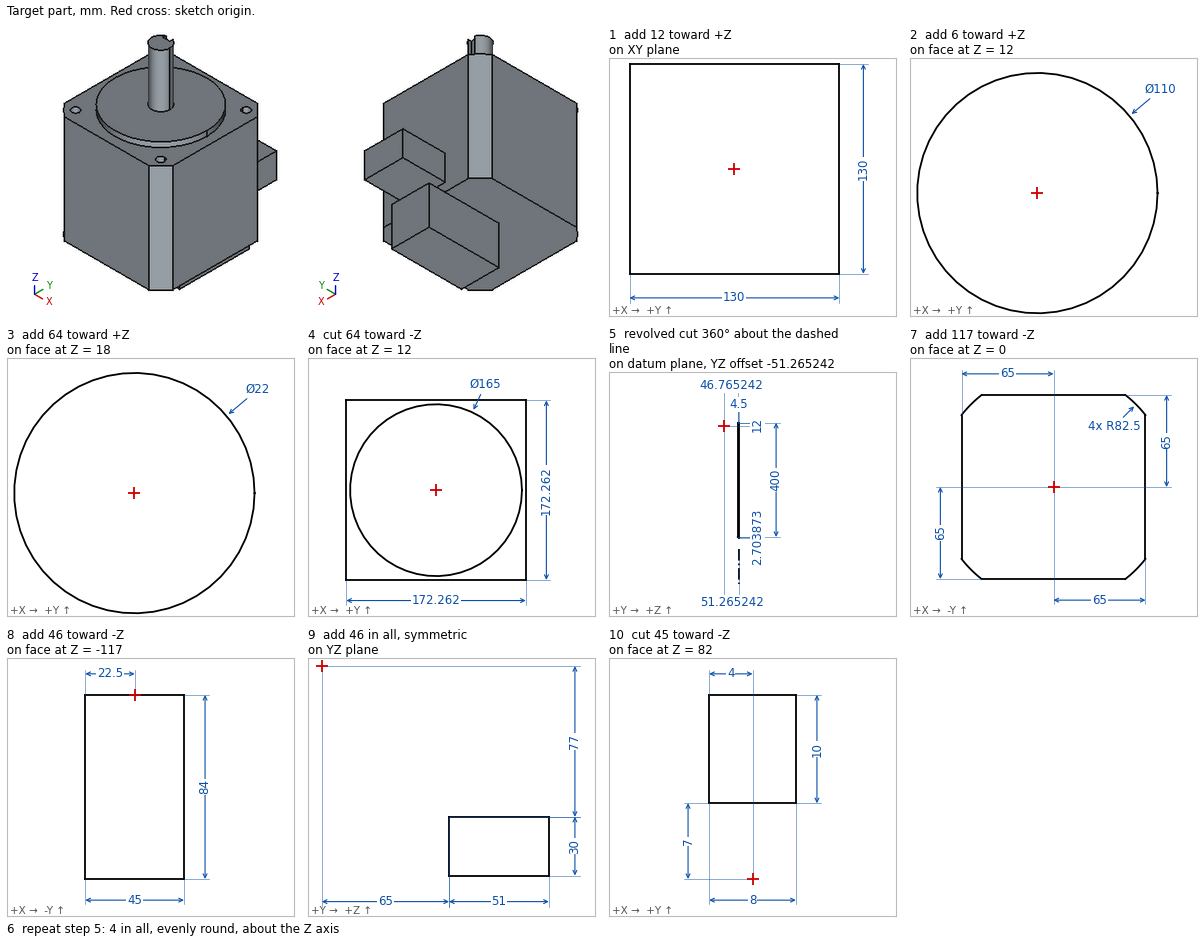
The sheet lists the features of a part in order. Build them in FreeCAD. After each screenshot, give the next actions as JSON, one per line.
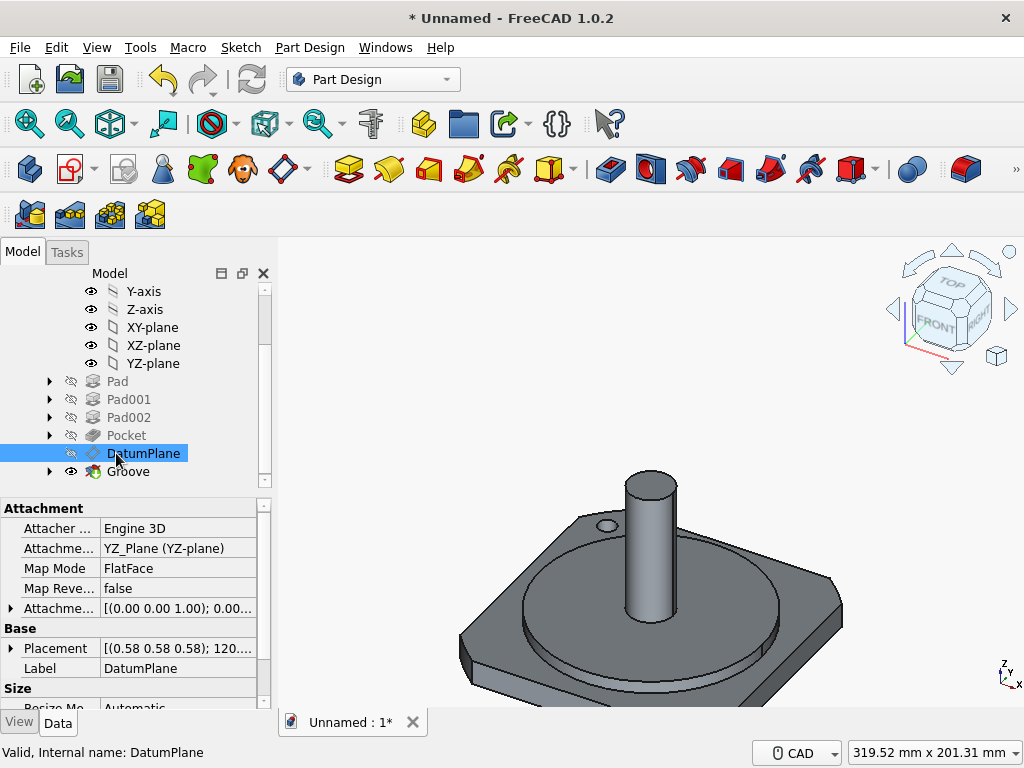
{"action": "left_click", "coordinate": [30, 124]}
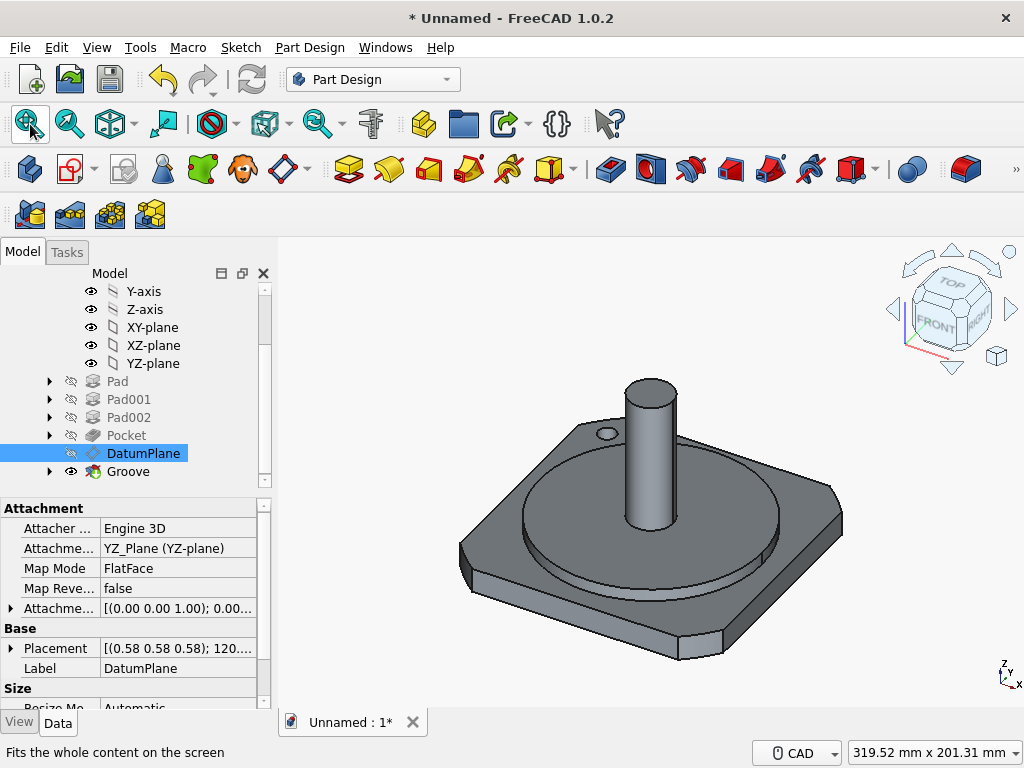
{"action": "left_click", "coordinate": [116, 471]}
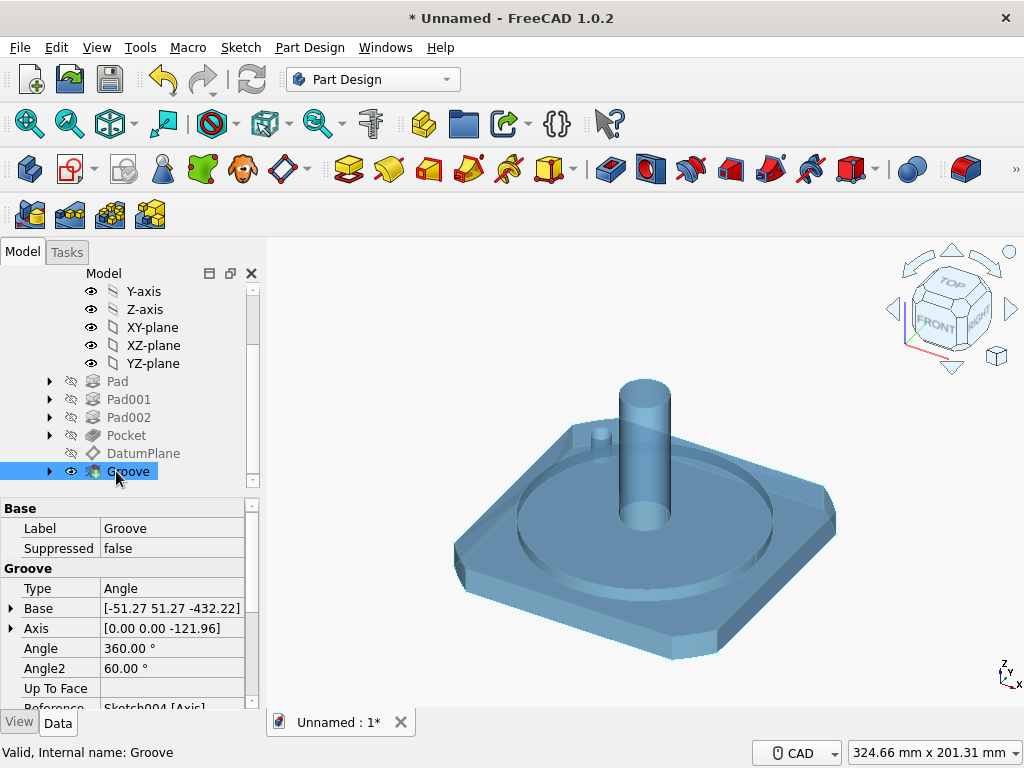
{"action": "left_click", "coordinate": [110, 214]}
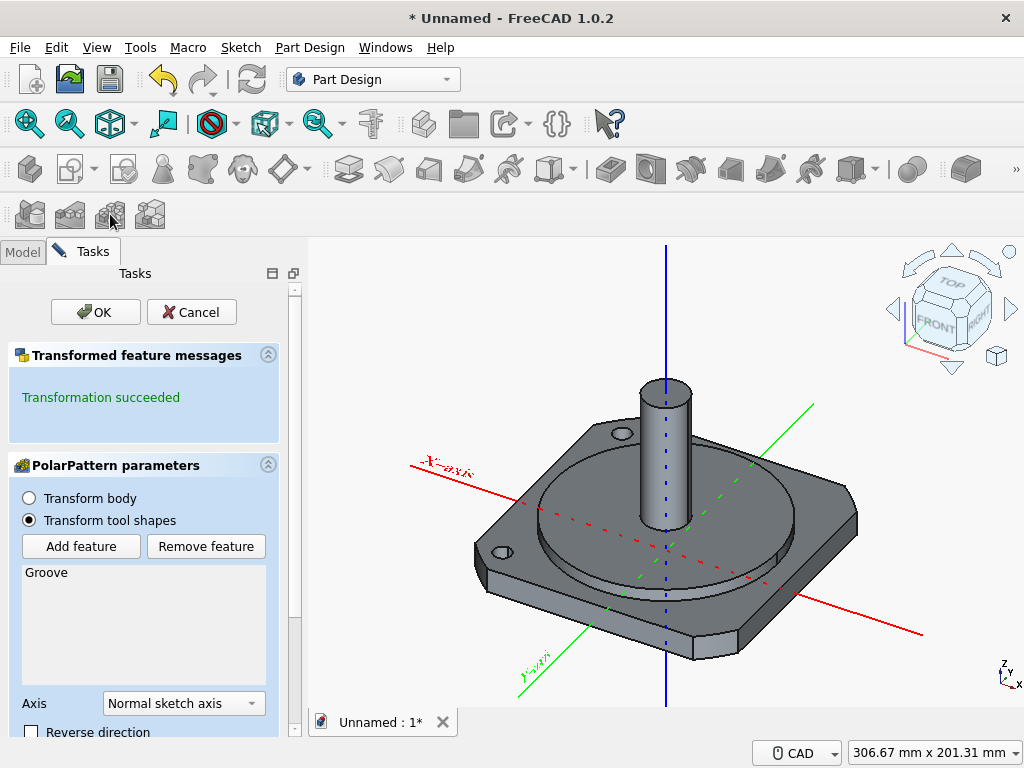
{"action": "left_click", "coordinate": [184, 704]}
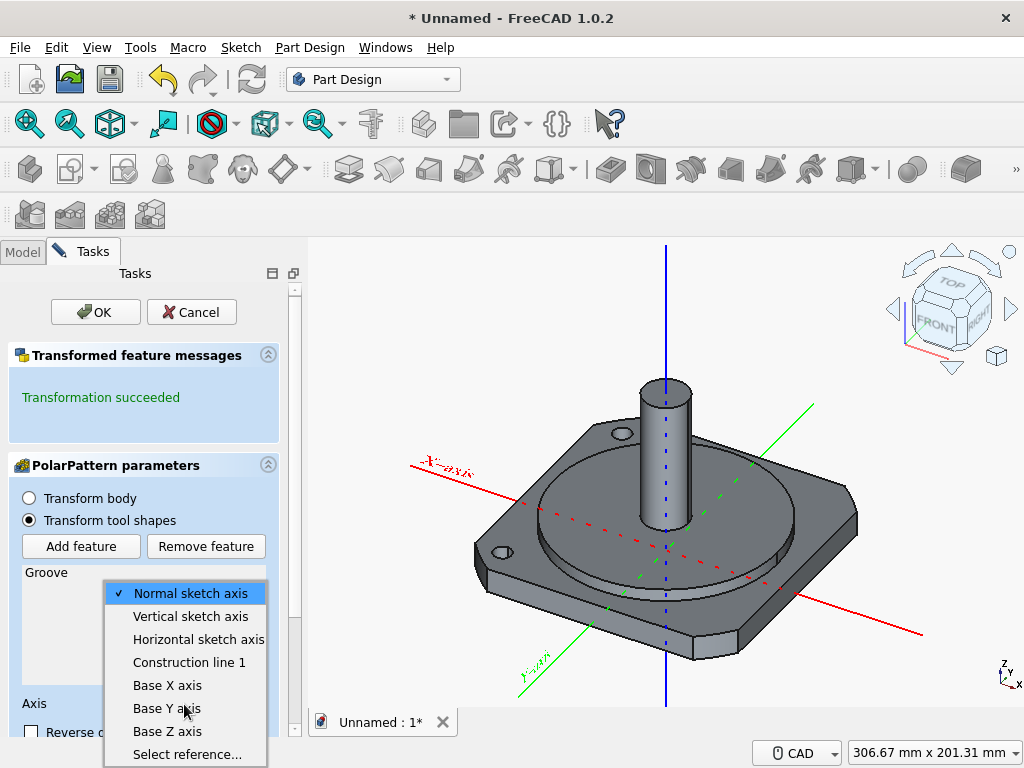
{"action": "left_click", "coordinate": [184, 732]}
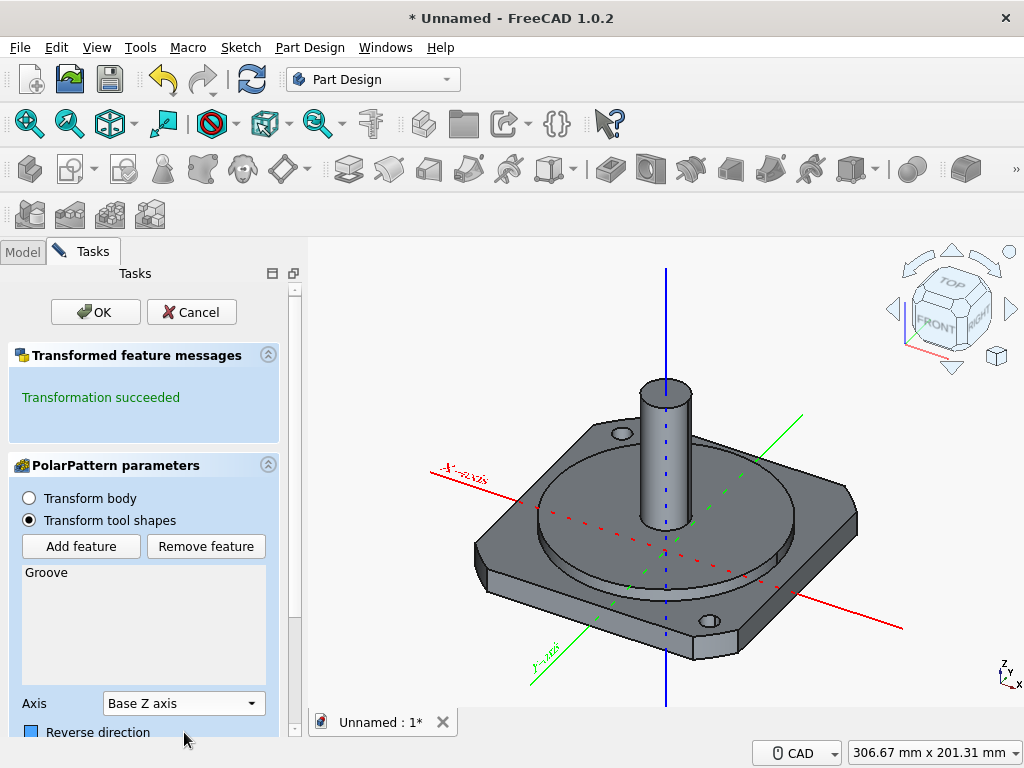
{"action": "scroll", "coordinate": [295, 510], "scroll_direction": "down", "scroll_amount": 3}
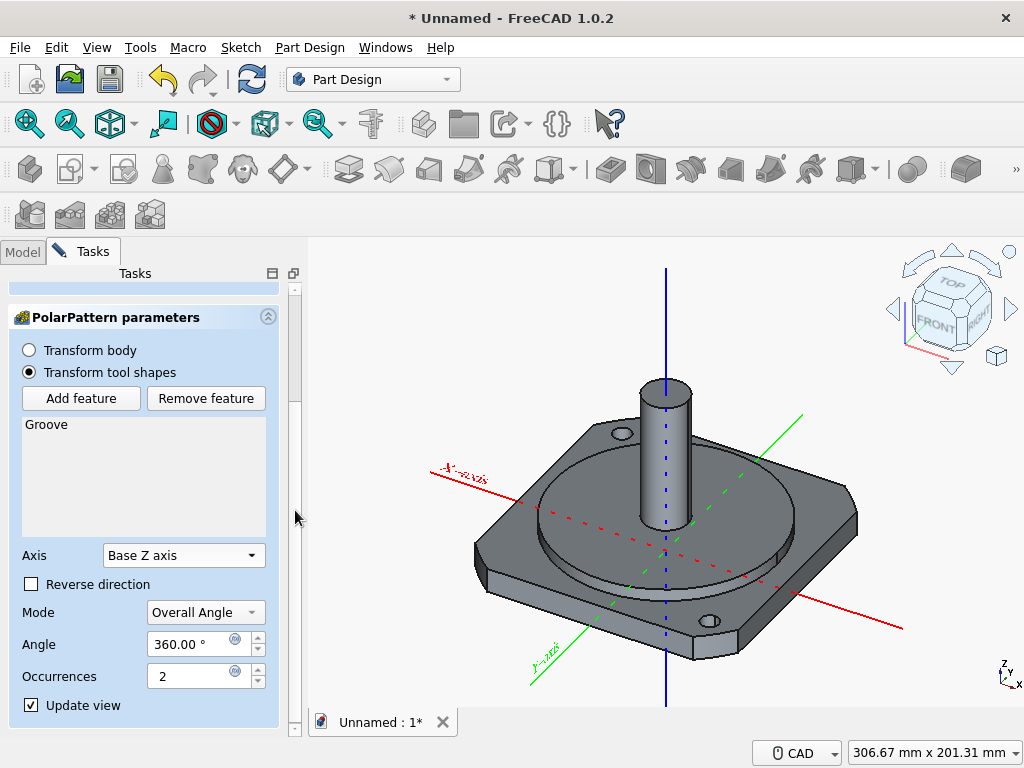
{"action": "triple_click", "coordinate": [198, 676]}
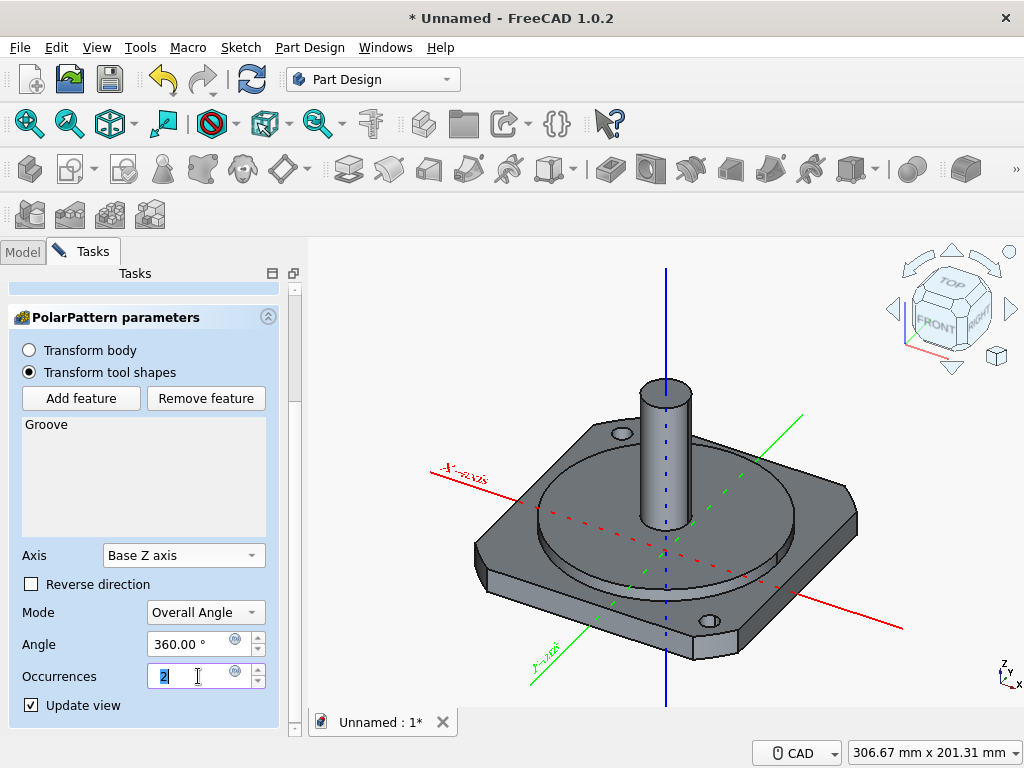
{"action": "type", "text": "4"}
{"action": "key", "text": "Tab"}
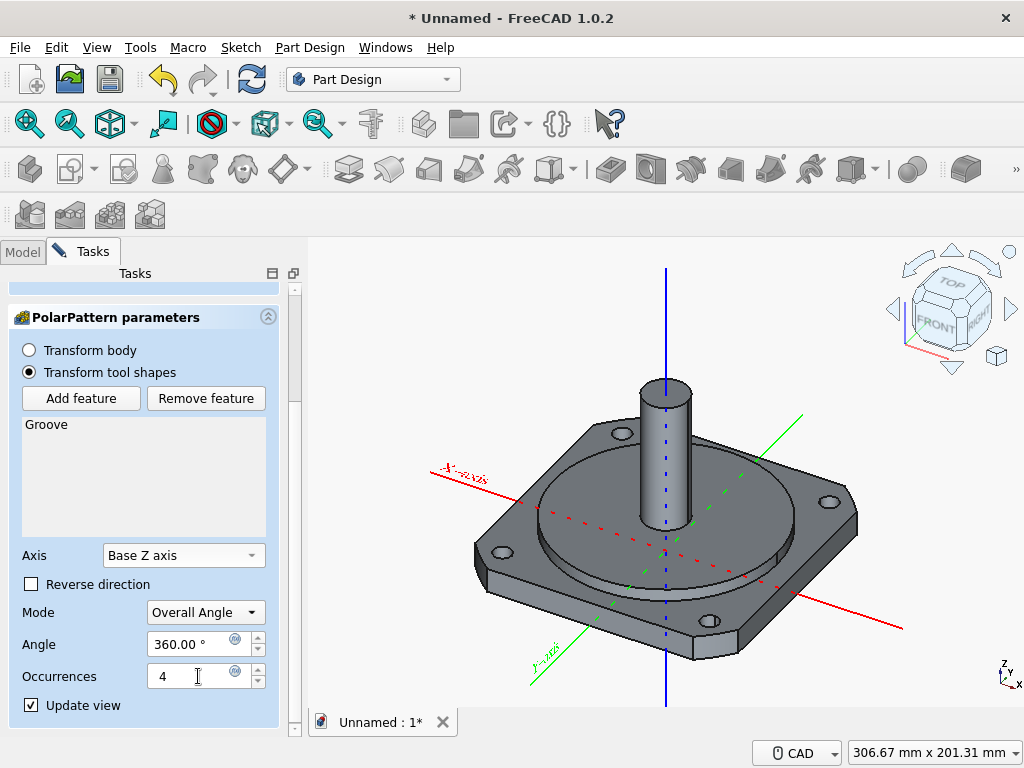
{"action": "scroll", "coordinate": [295, 510], "scroll_direction": "up", "scroll_amount": 4}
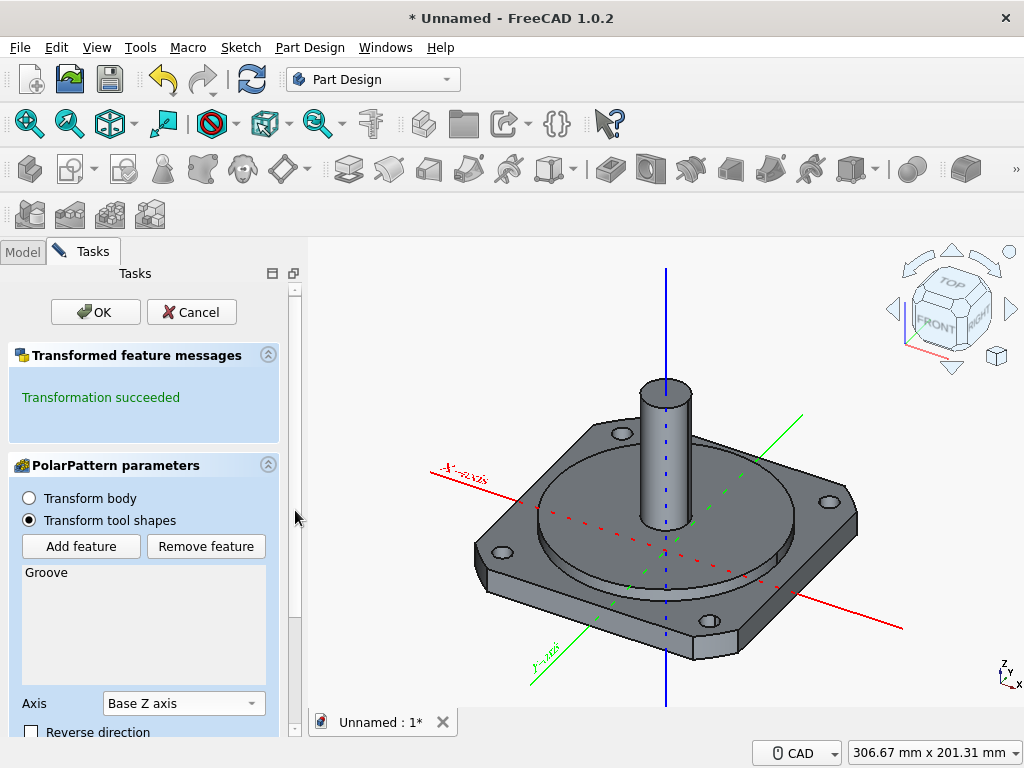
{"action": "left_click", "coordinate": [96, 312]}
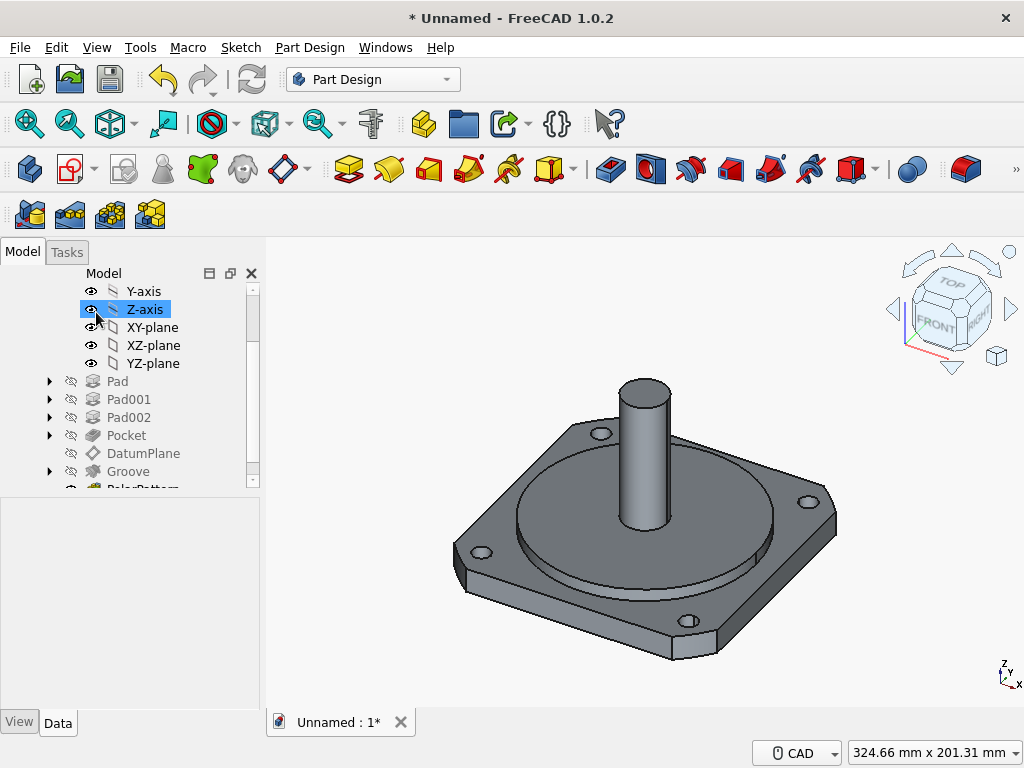
{"action": "key", "text": "5"}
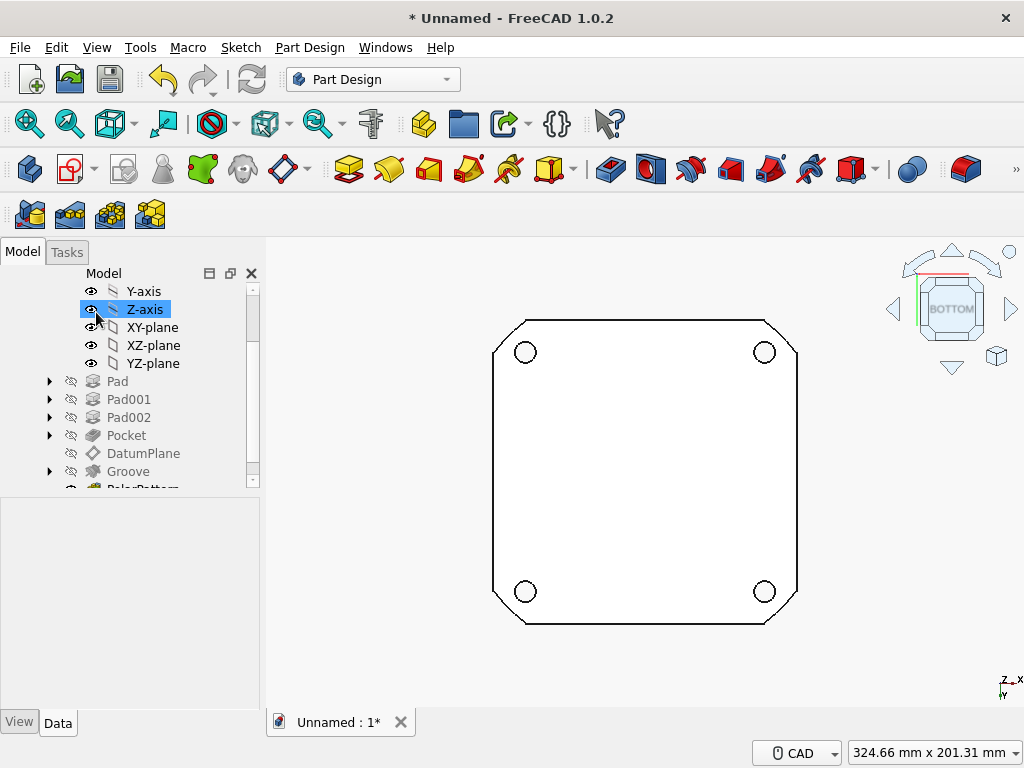
{"action": "left_click", "coordinate": [645, 471]}